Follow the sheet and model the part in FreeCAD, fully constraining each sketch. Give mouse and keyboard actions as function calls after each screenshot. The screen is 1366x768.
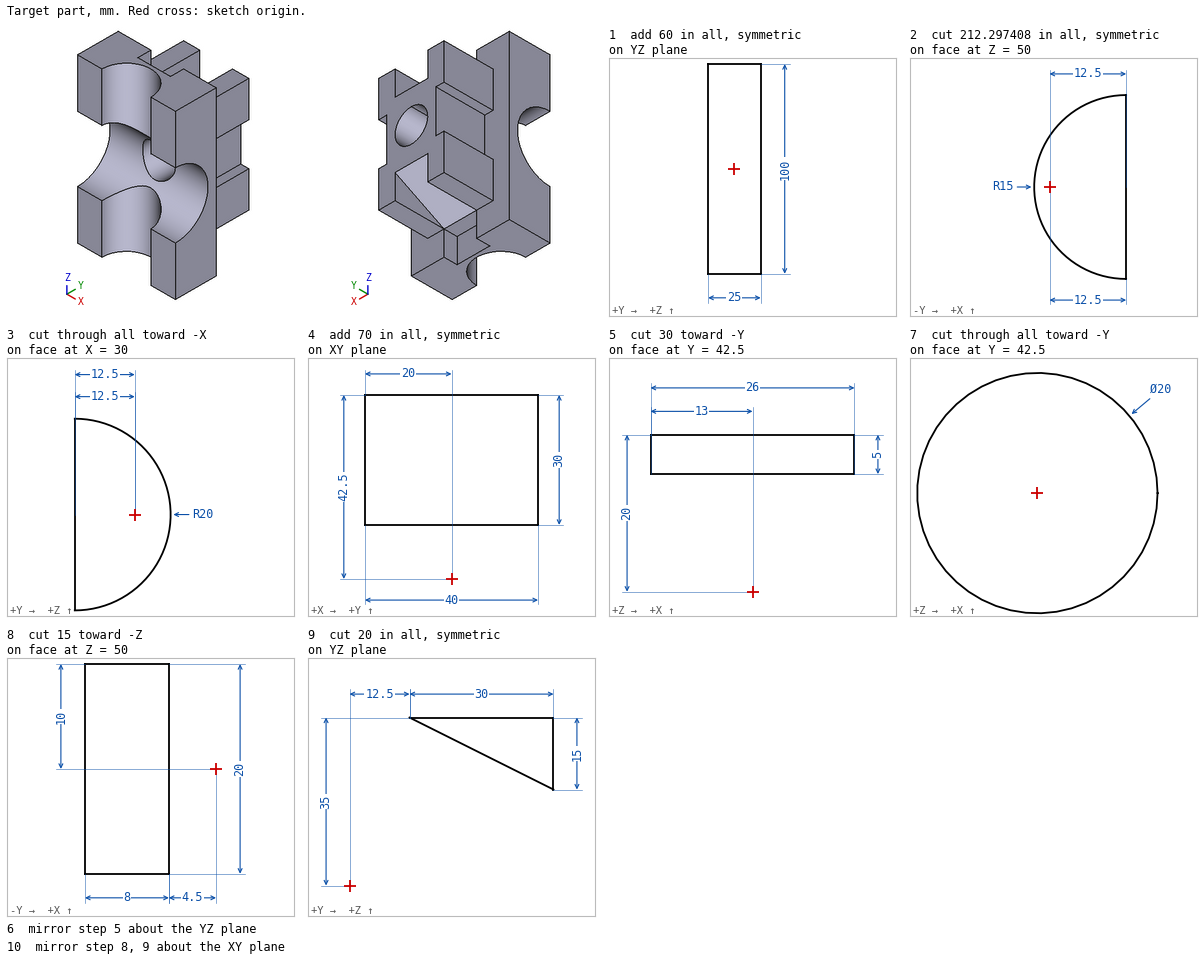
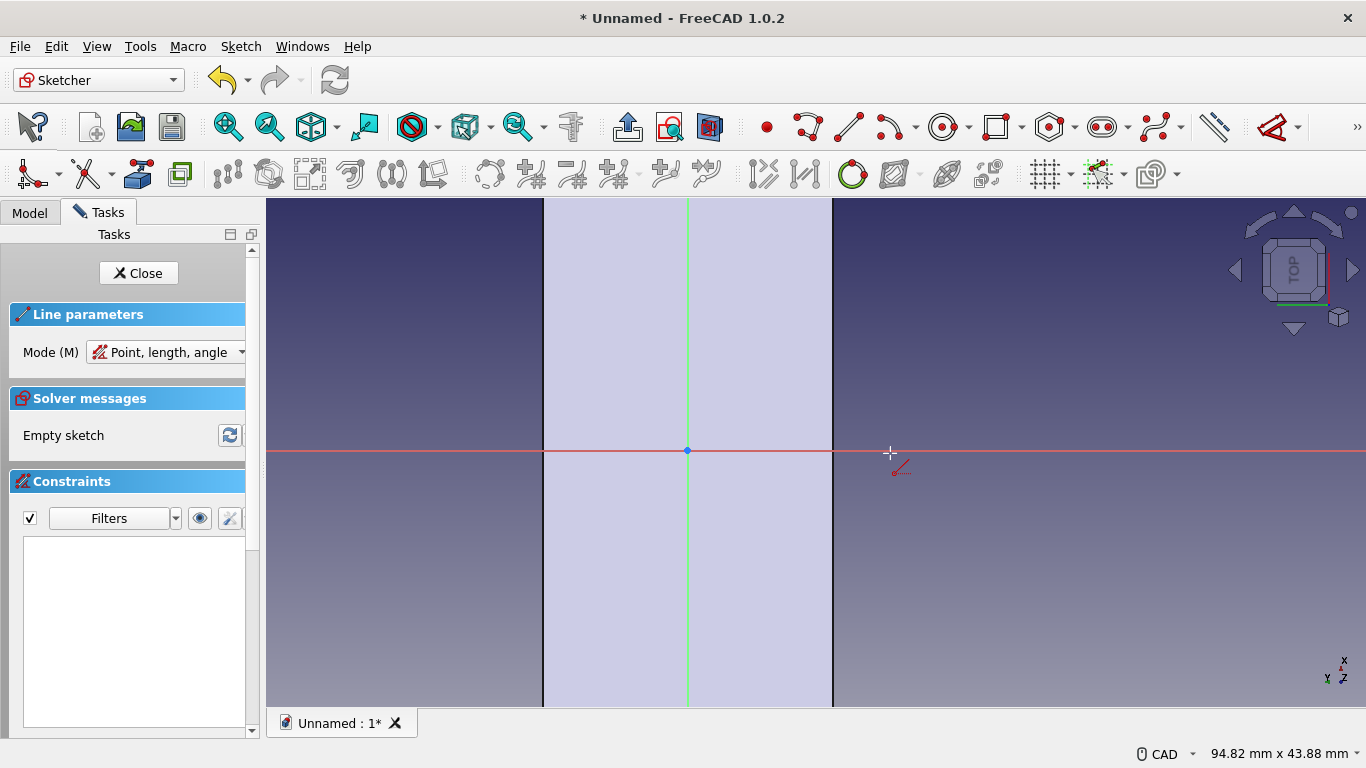
click(833, 625)
click(833, 277)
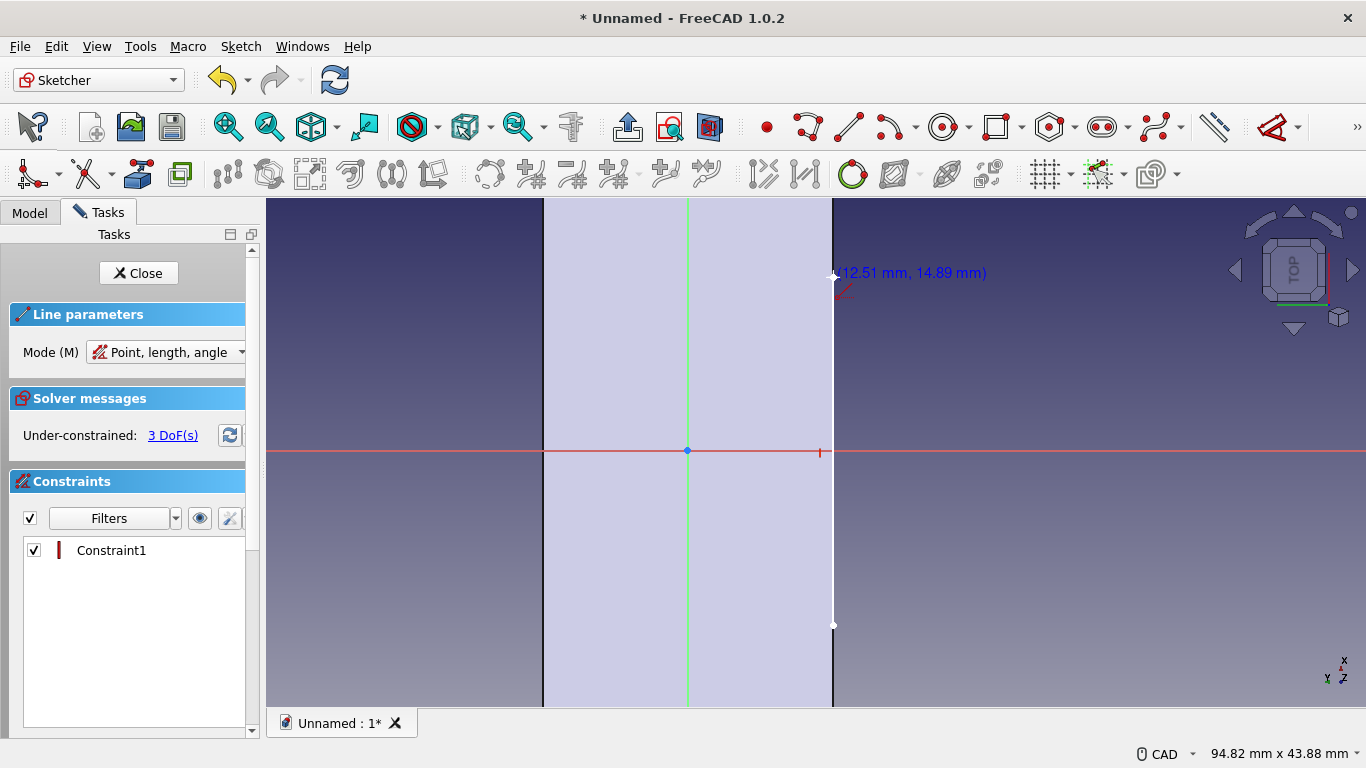
key(g)
key(3)
key(a)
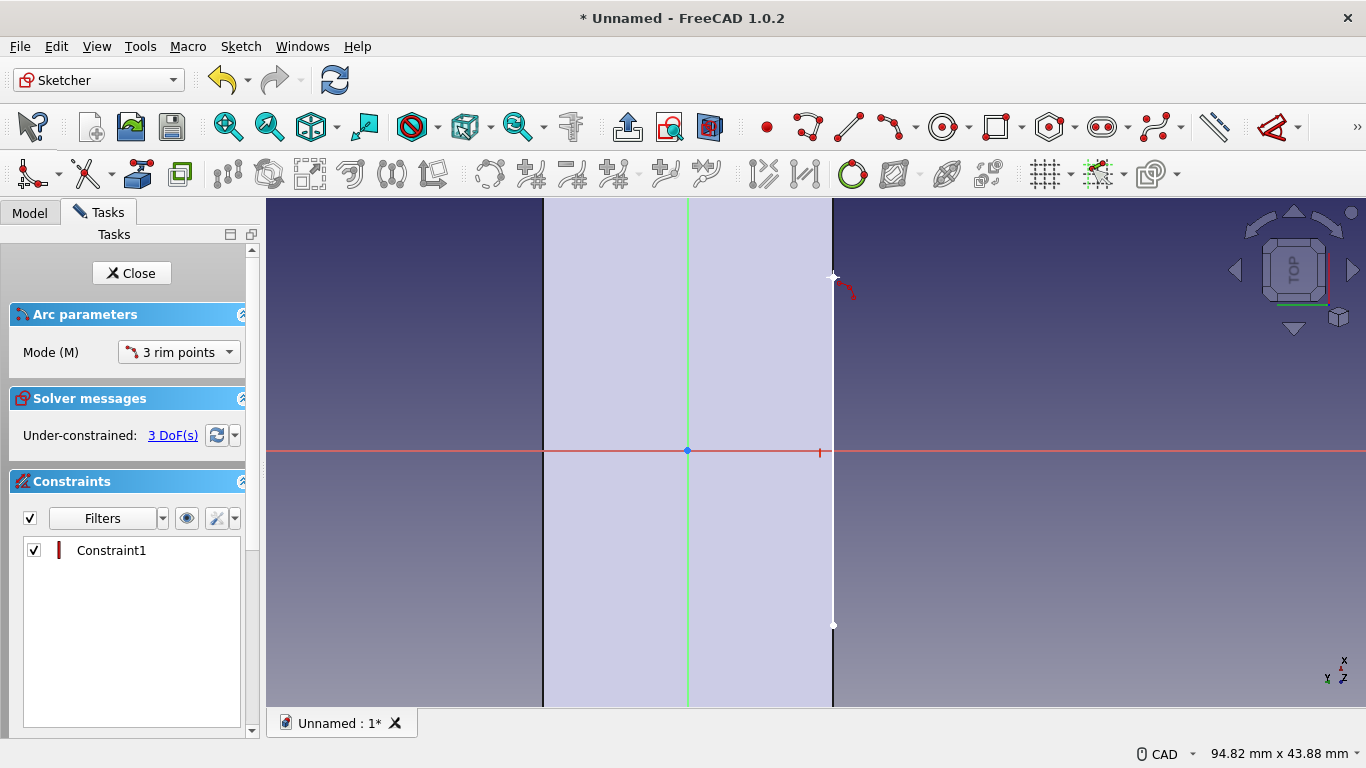
click(833, 278)
click(833, 626)
click(667, 397)
key(Escape)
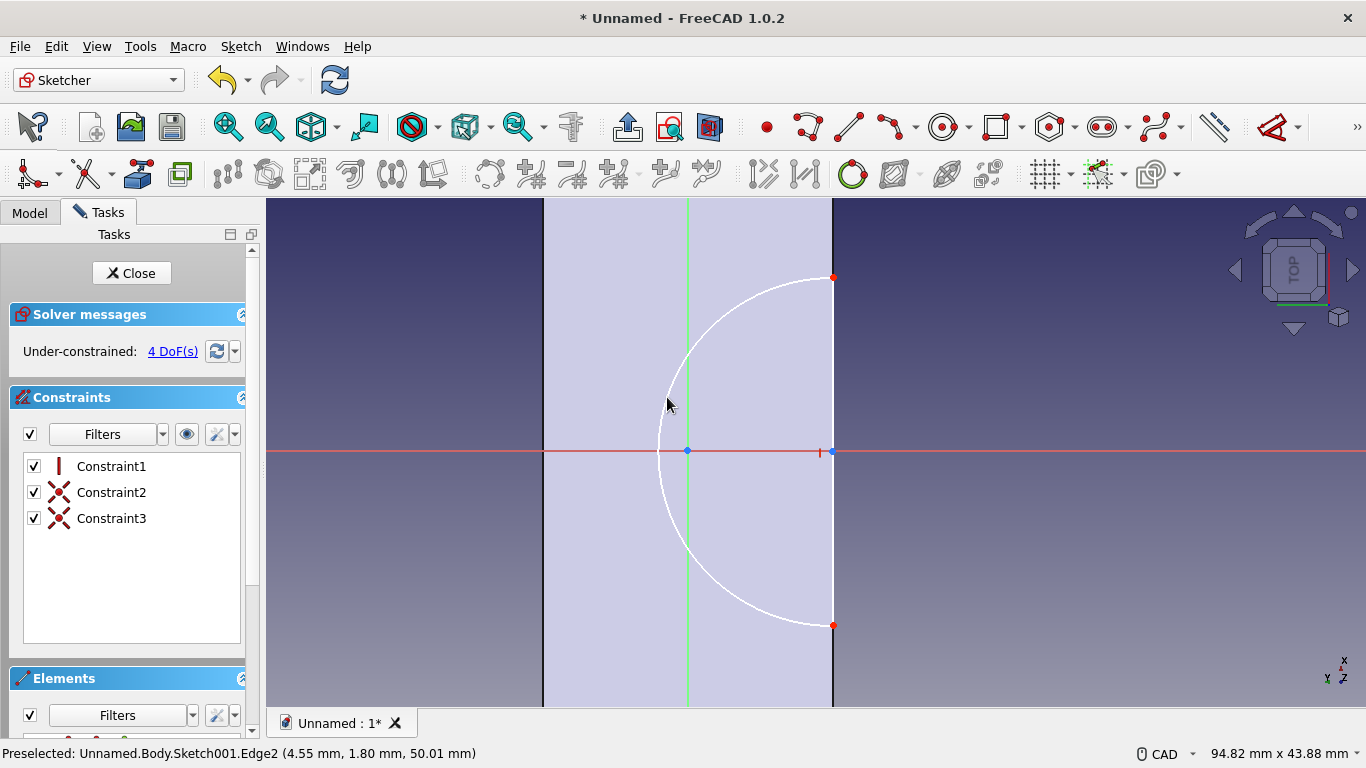
click(832, 452)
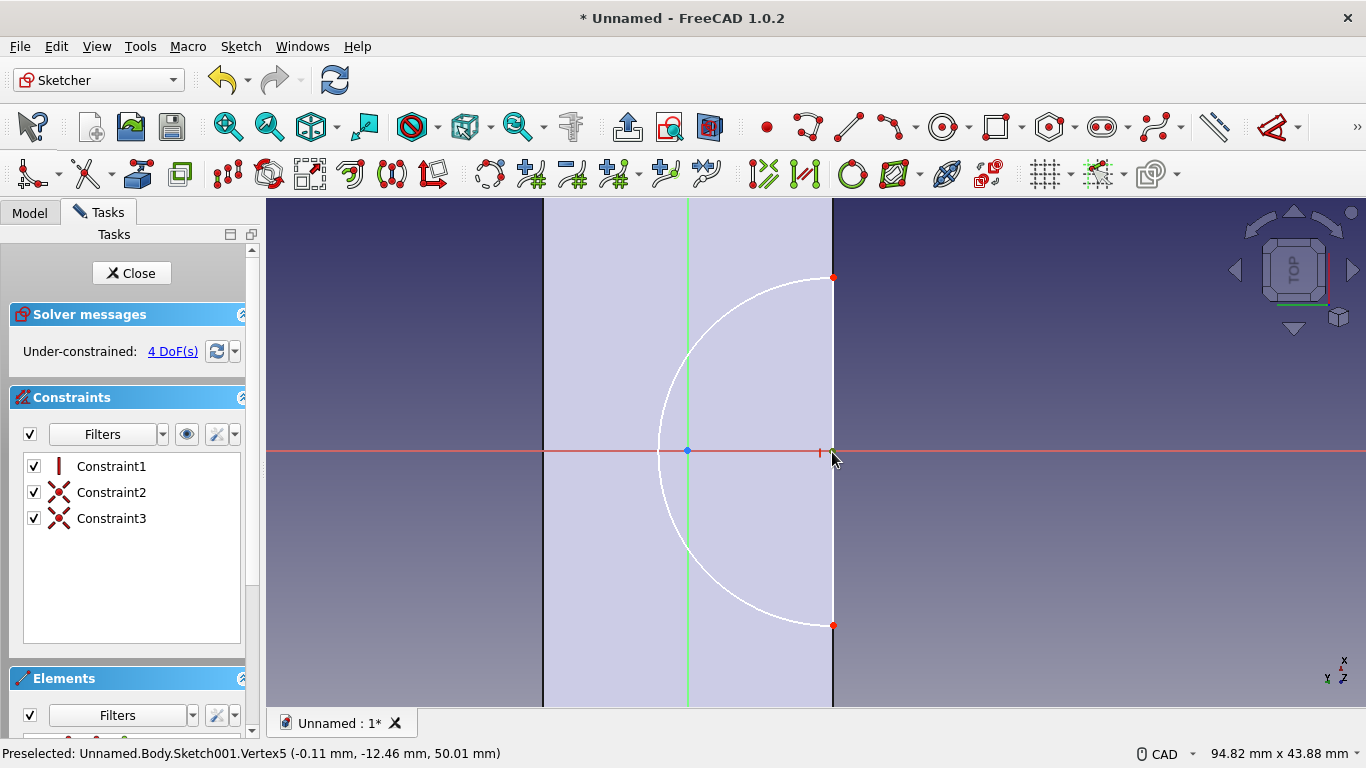
click(359, 451)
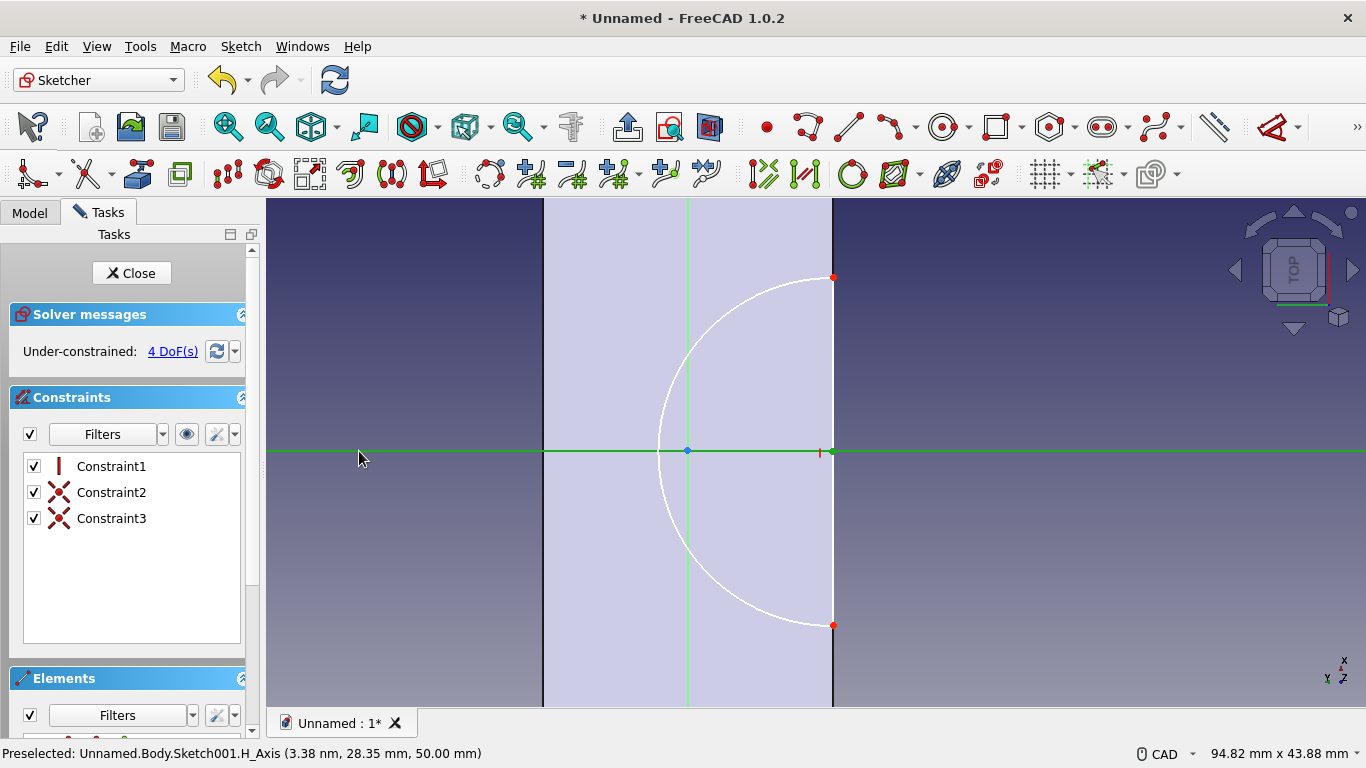
key(c)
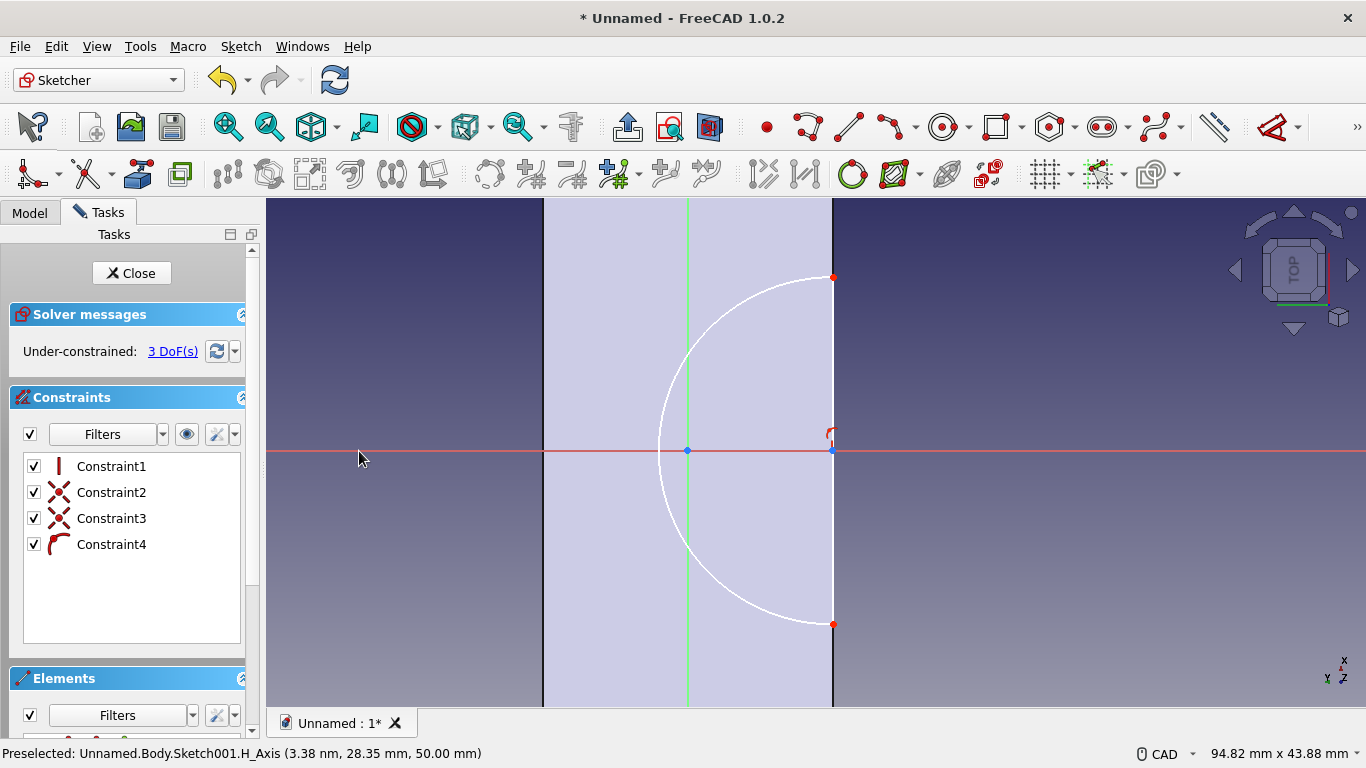
click(659, 451)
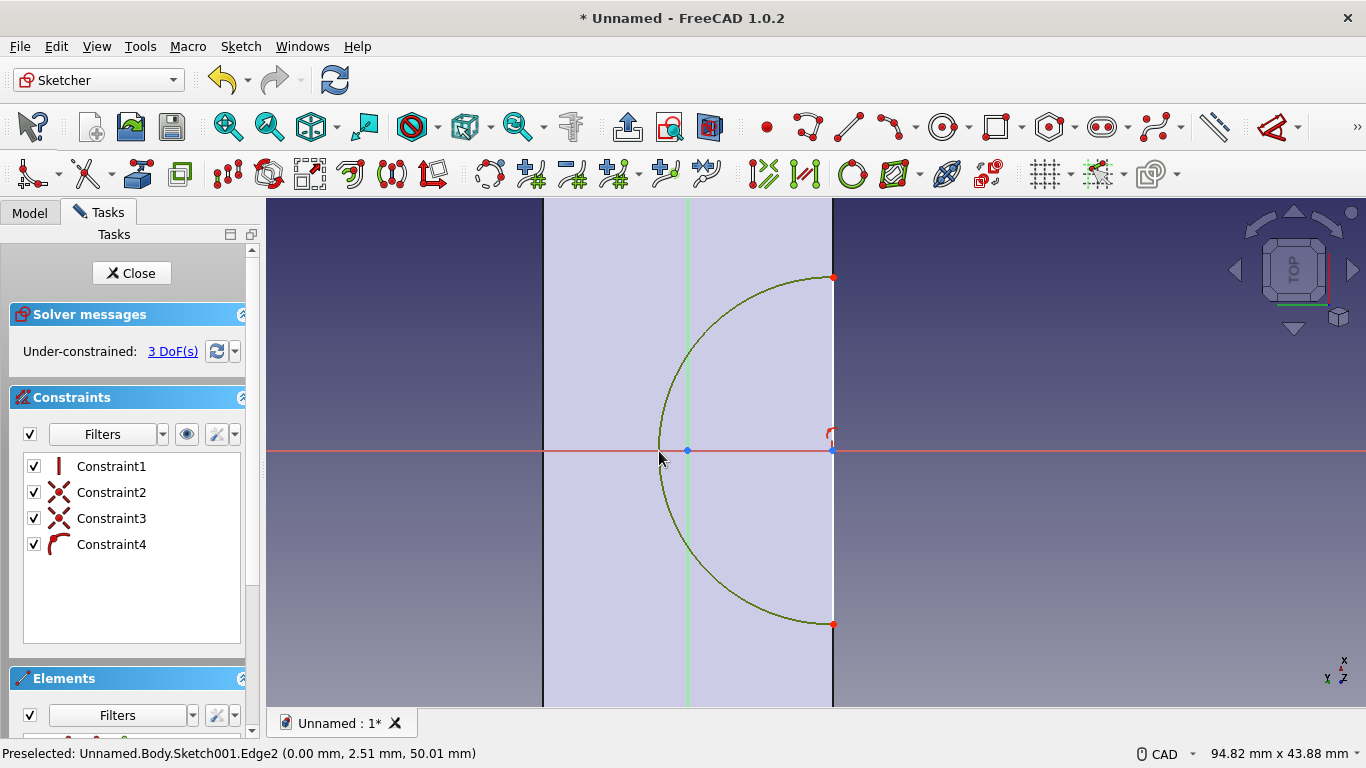
key(k)
key(r)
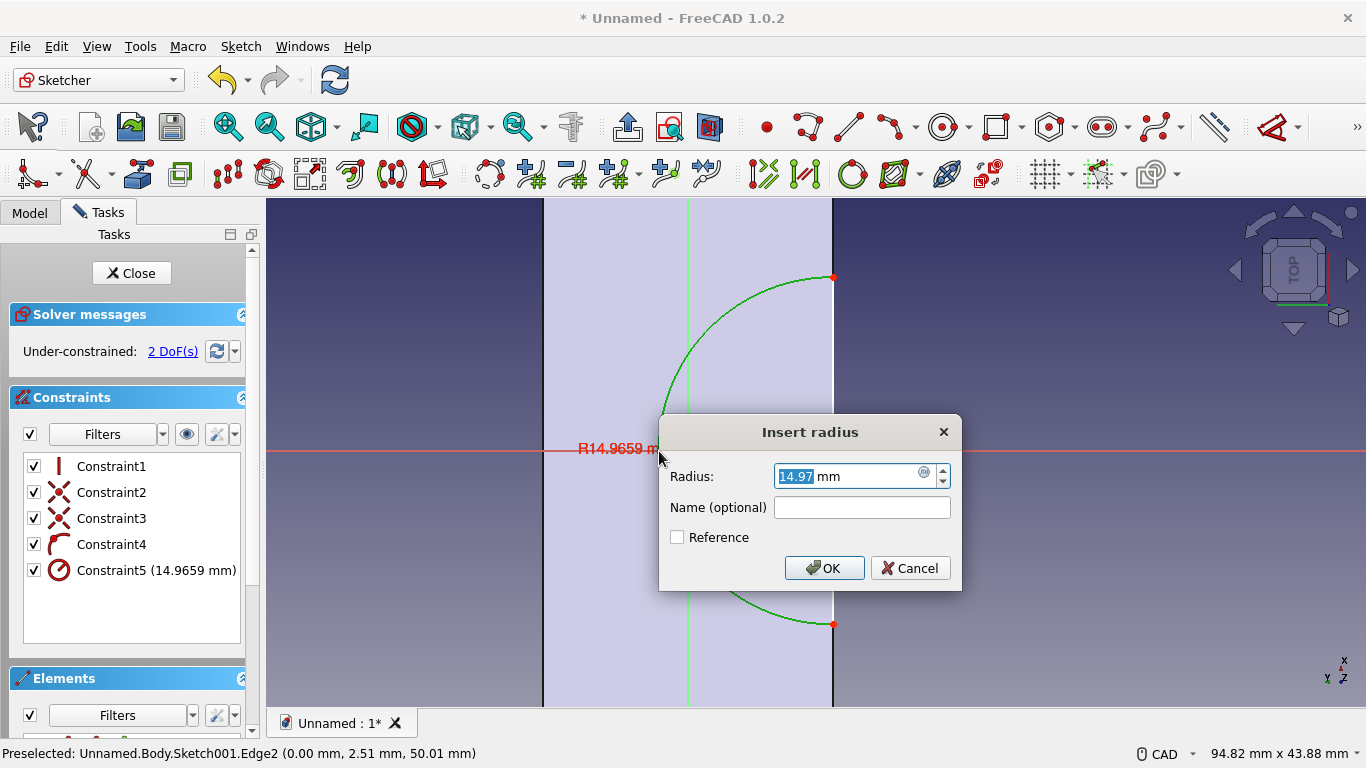
text(15)
key(Return)